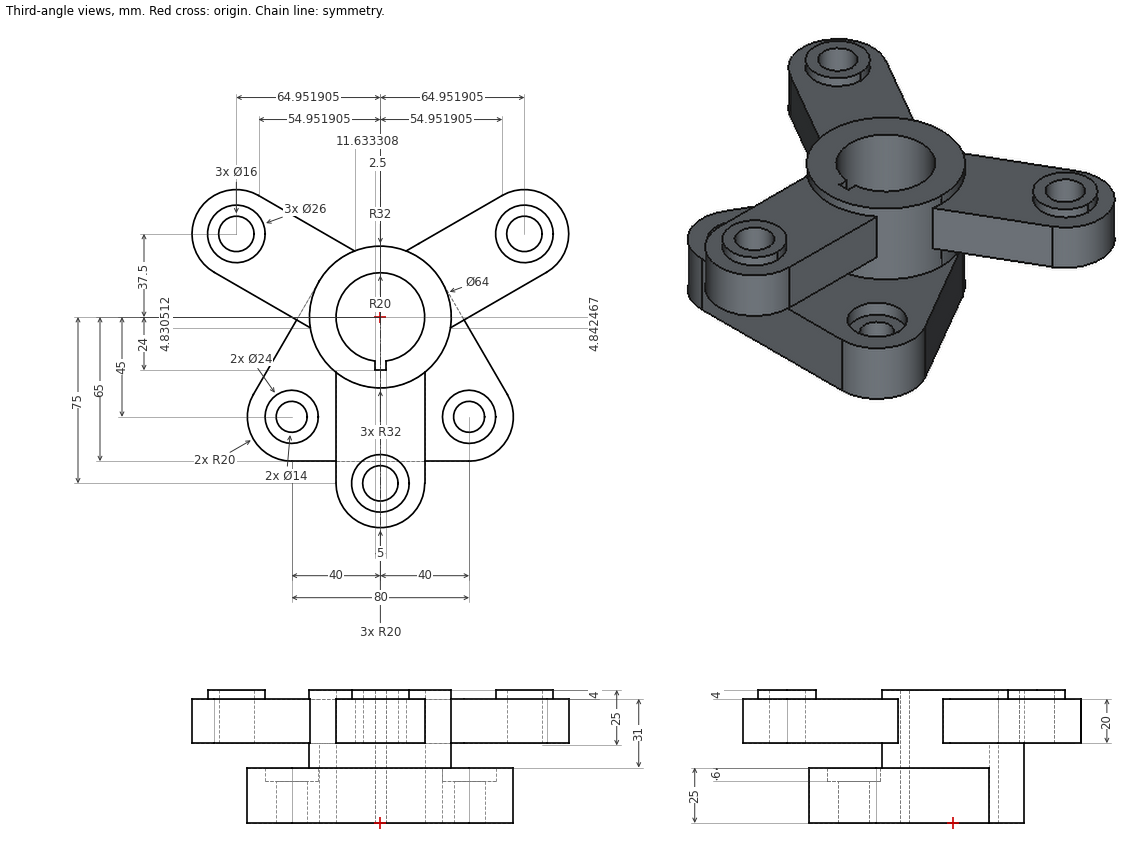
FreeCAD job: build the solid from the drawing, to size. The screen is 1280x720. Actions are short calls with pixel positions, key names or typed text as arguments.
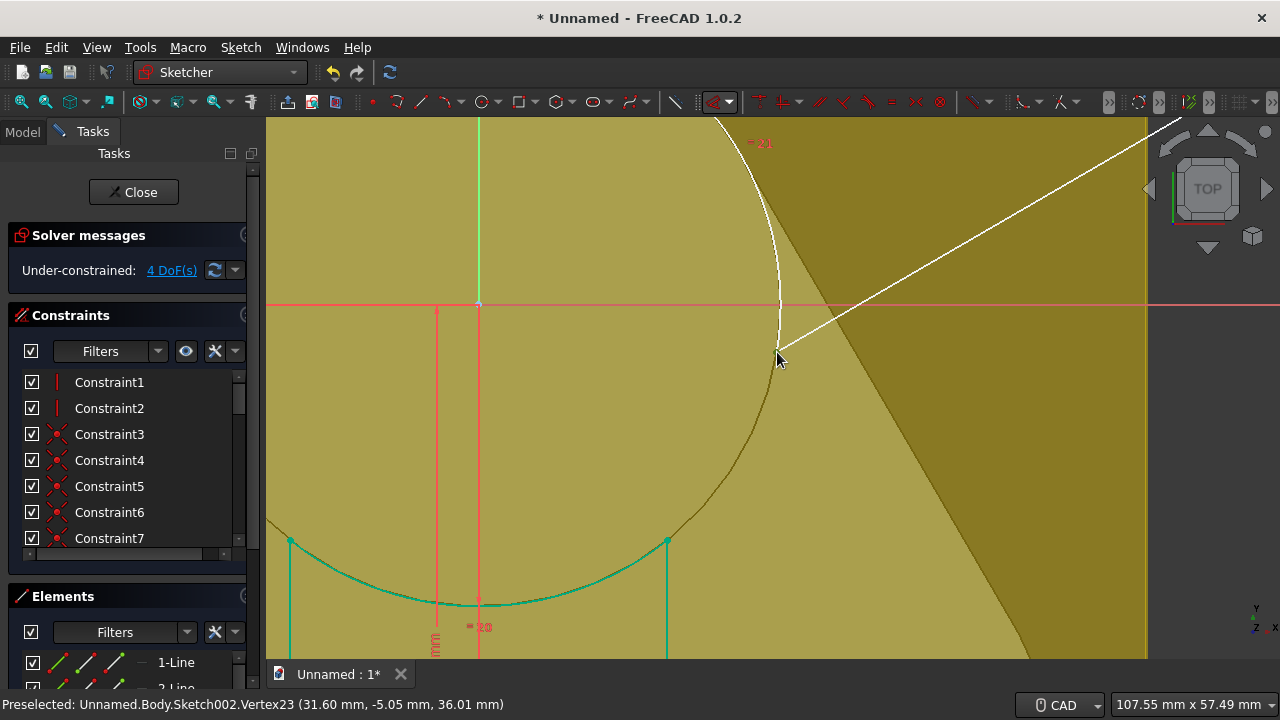
key(i)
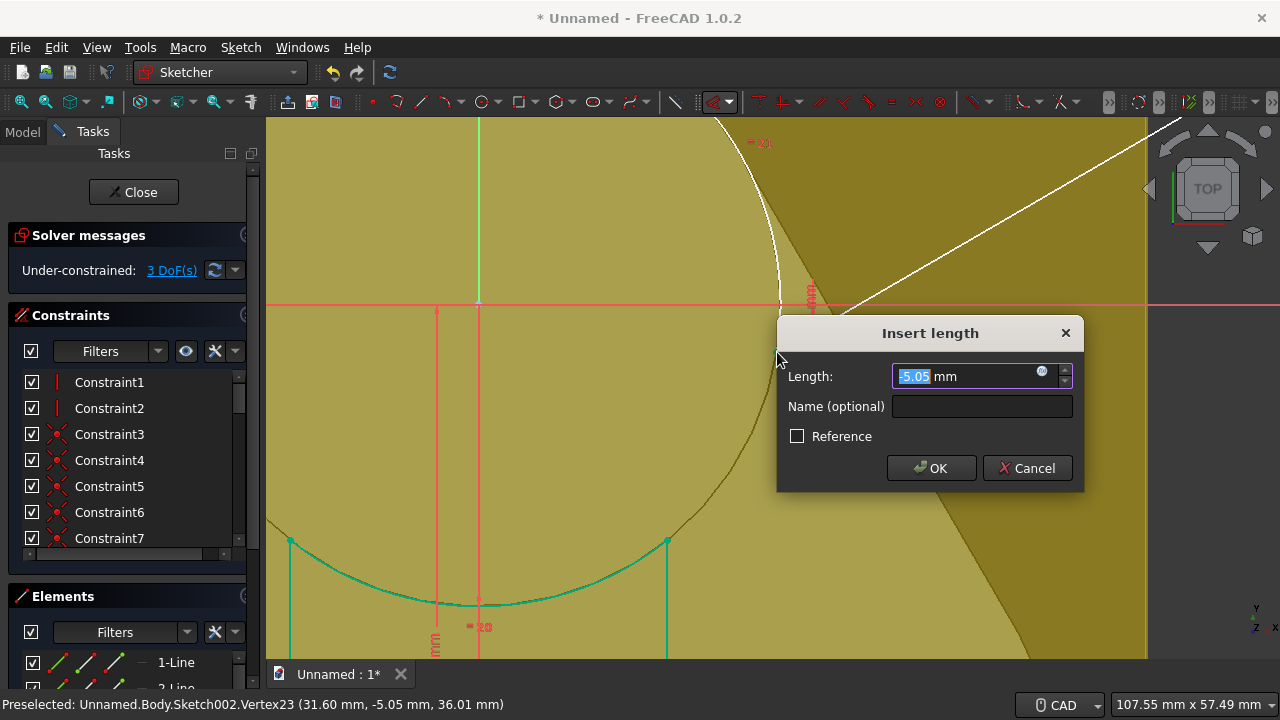
text(-4.842467)
key(Return)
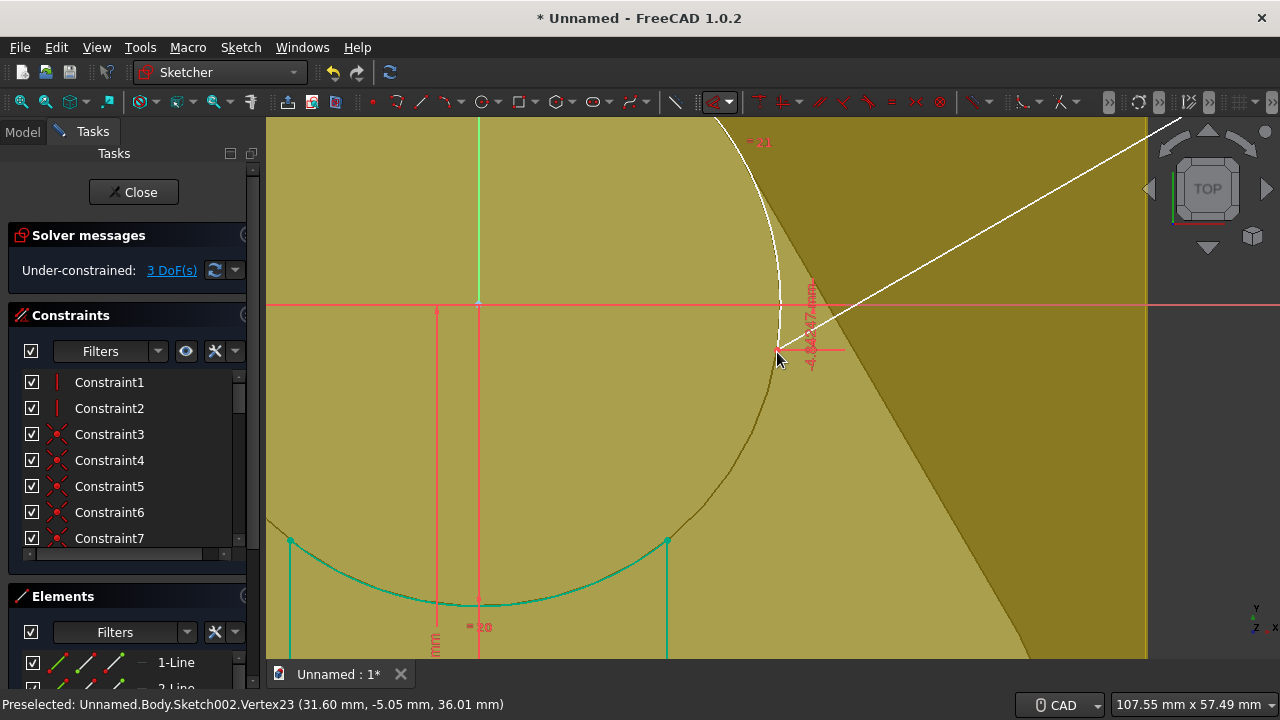
scroll(778, 353, down, 7)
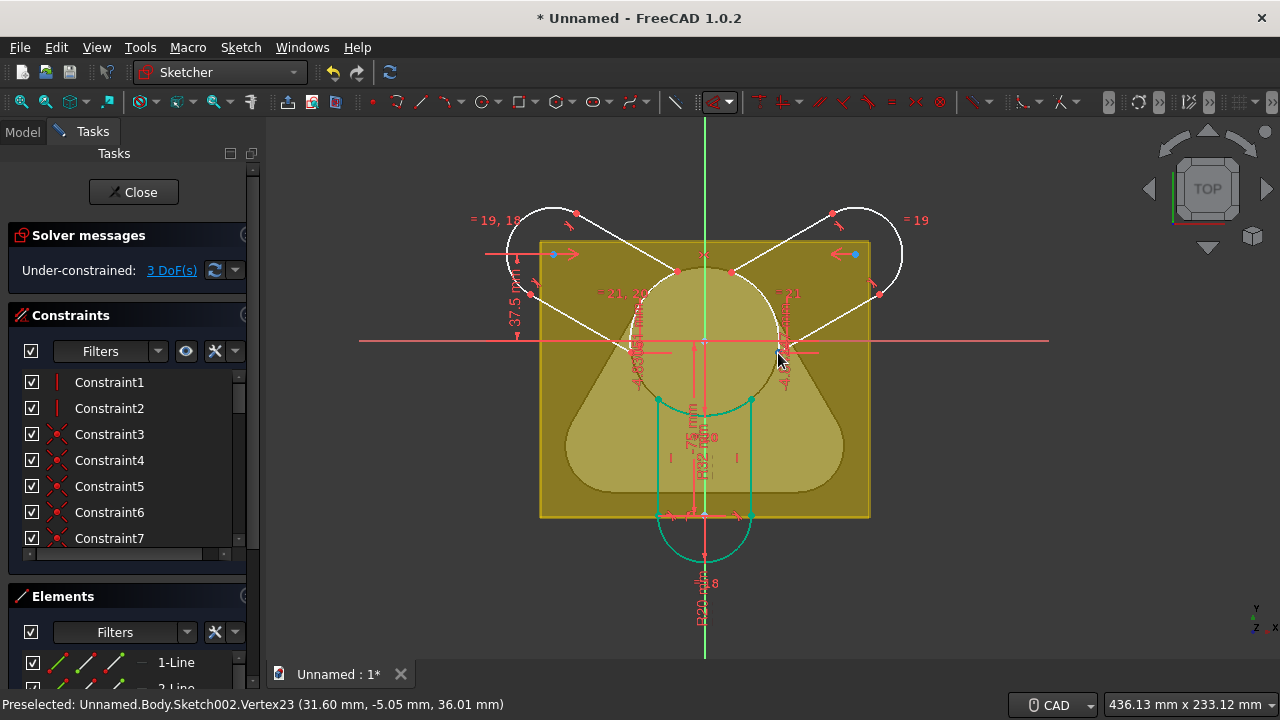
scroll(678, 272, up, 2)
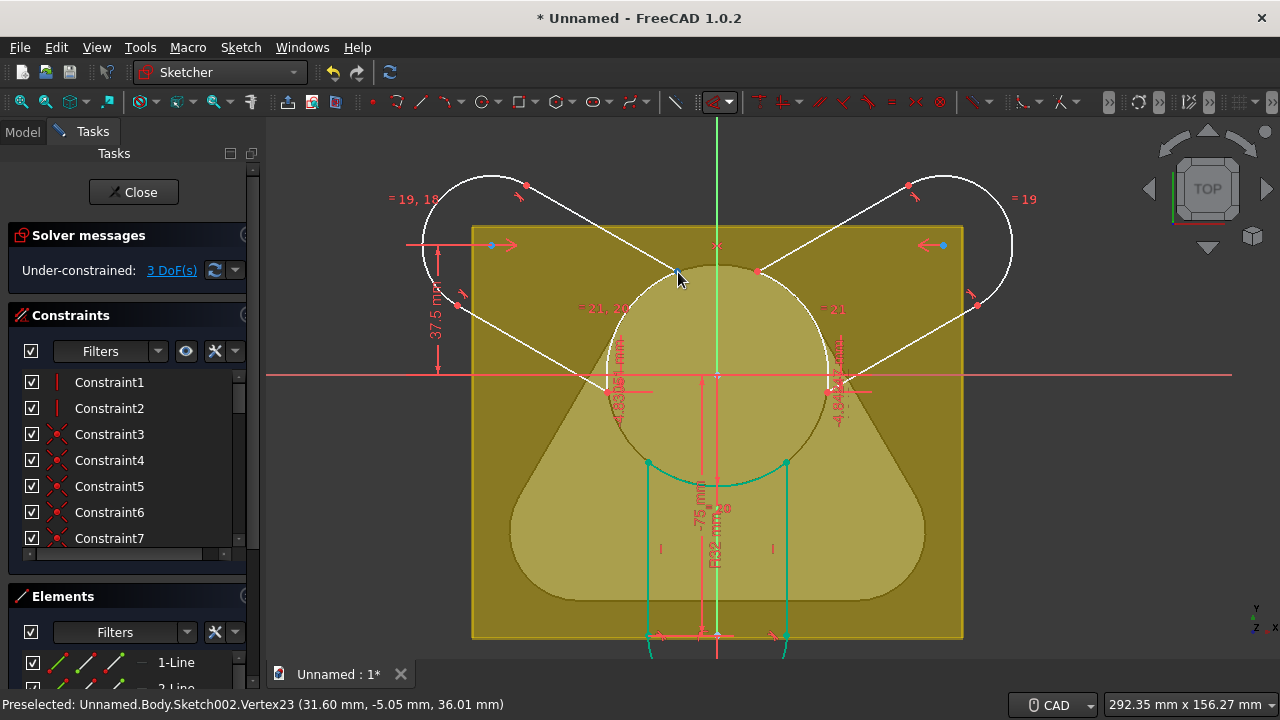
click(678, 272)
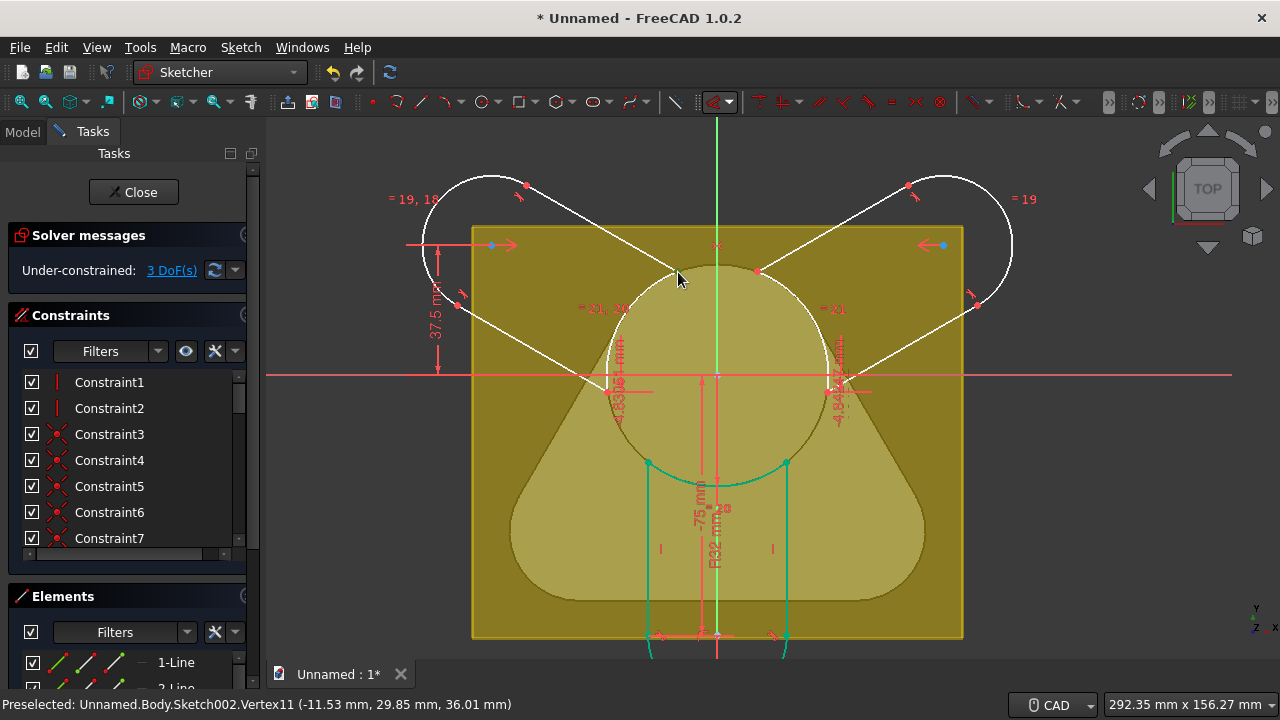
key(l)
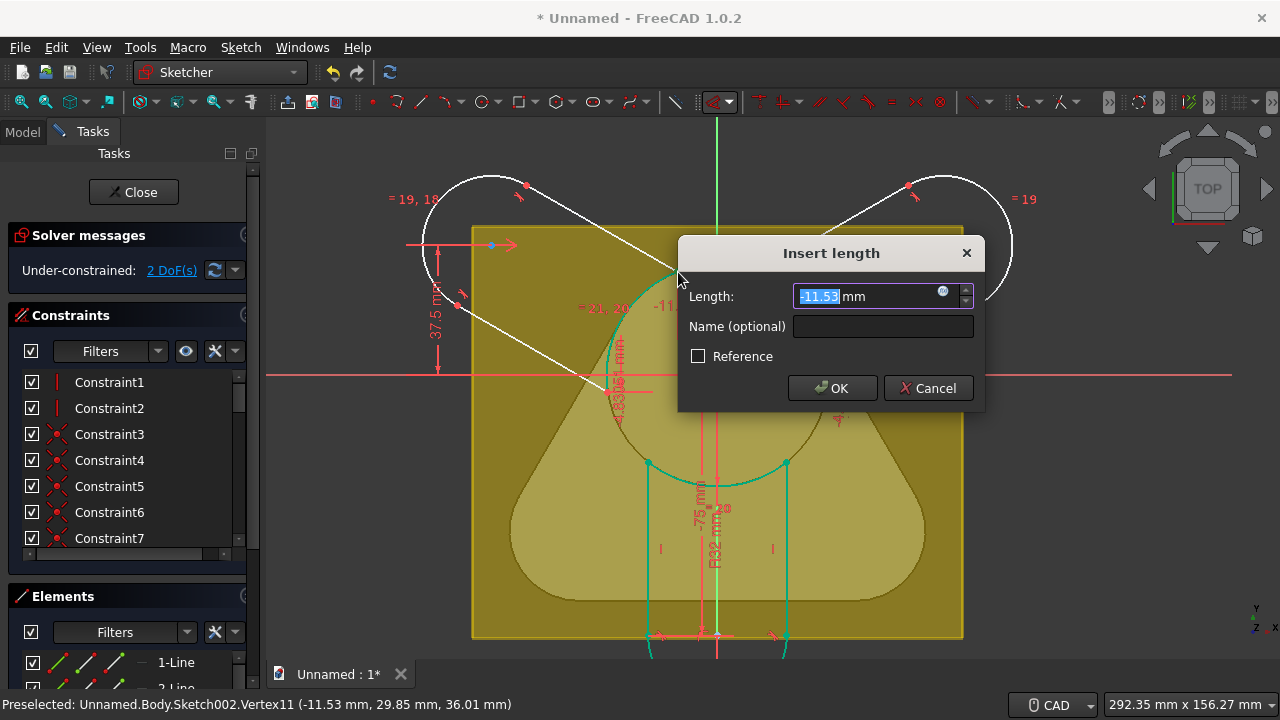
text(-11.633308)
key(Return)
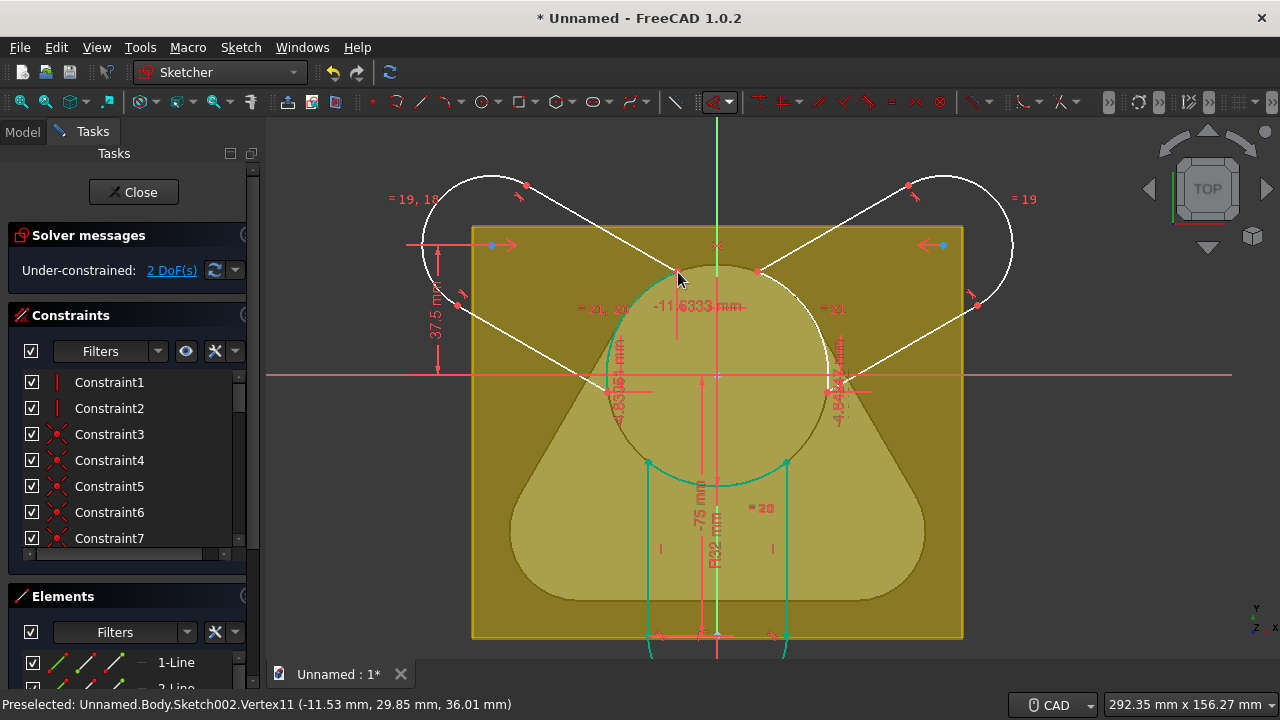
click(526, 185)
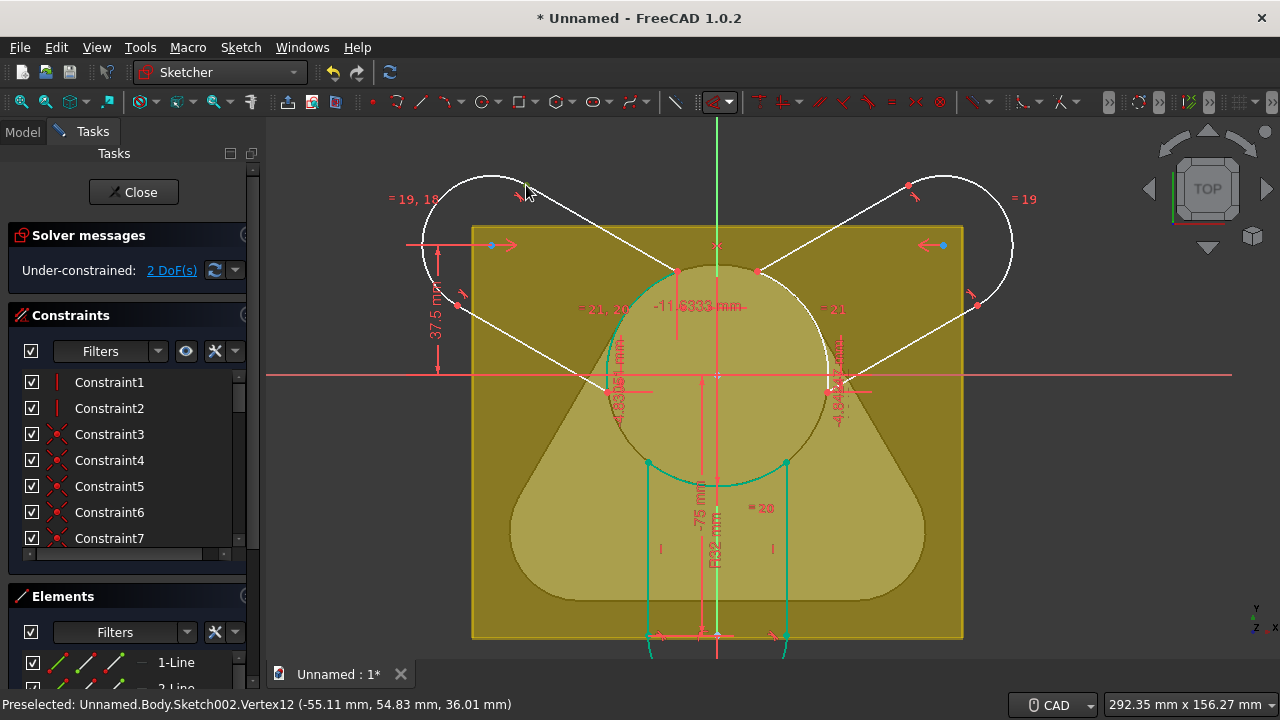
key(l)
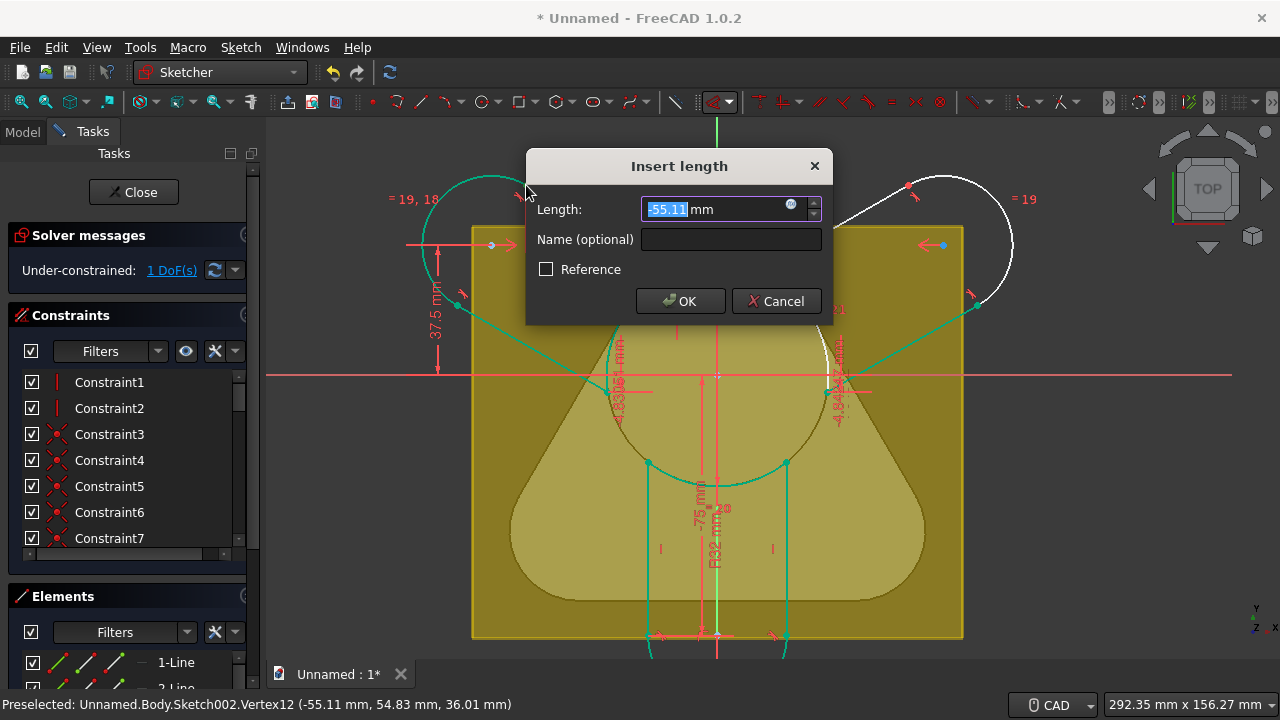
text(-54.951905)
key(Return)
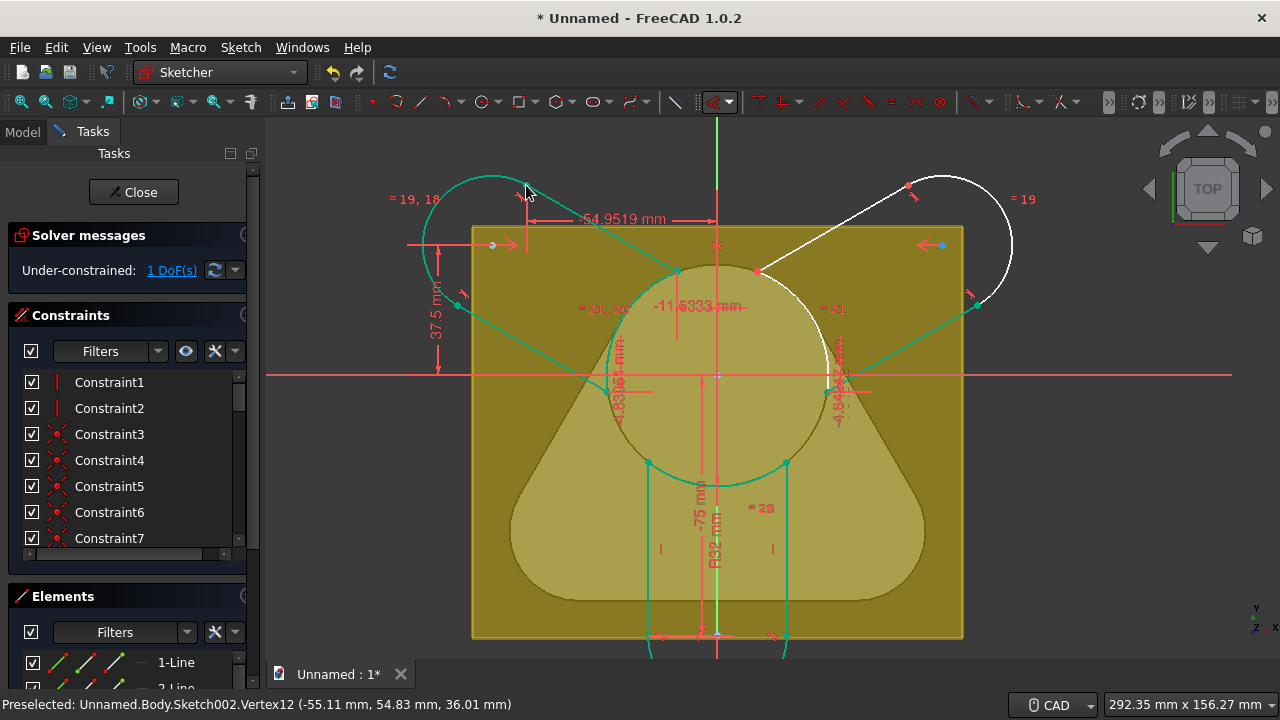
click(908, 185)